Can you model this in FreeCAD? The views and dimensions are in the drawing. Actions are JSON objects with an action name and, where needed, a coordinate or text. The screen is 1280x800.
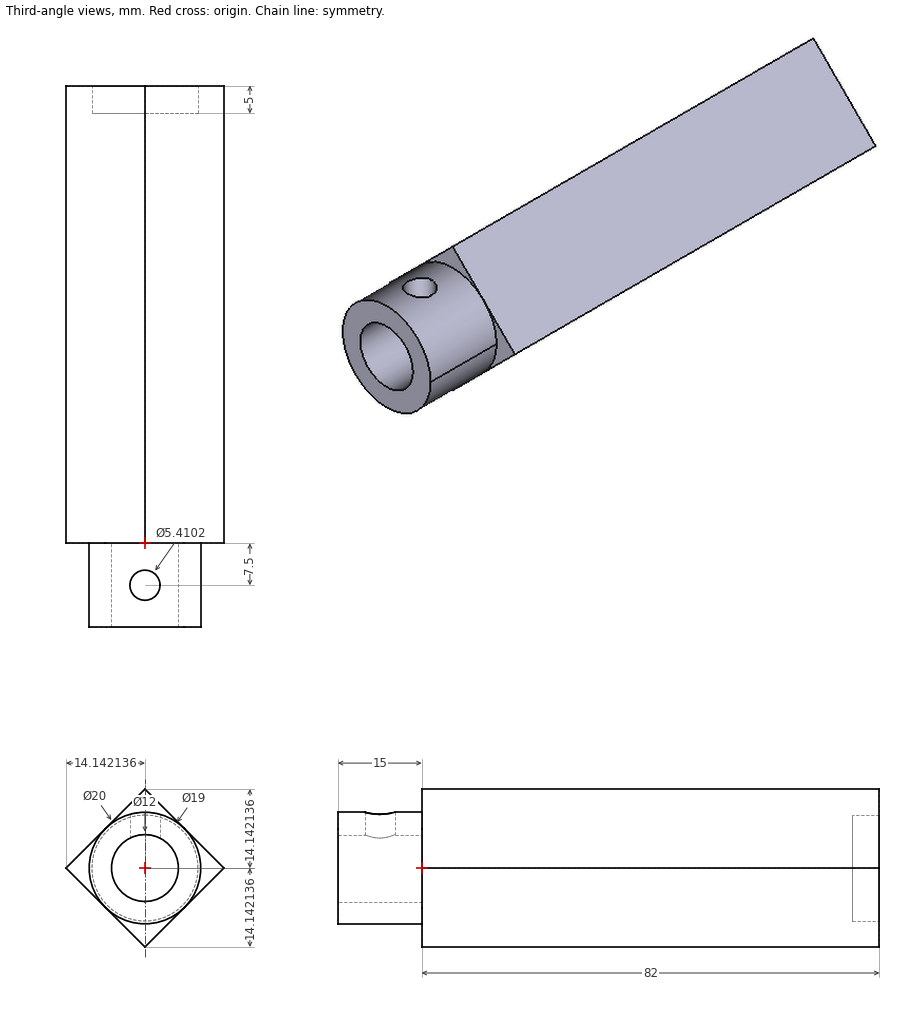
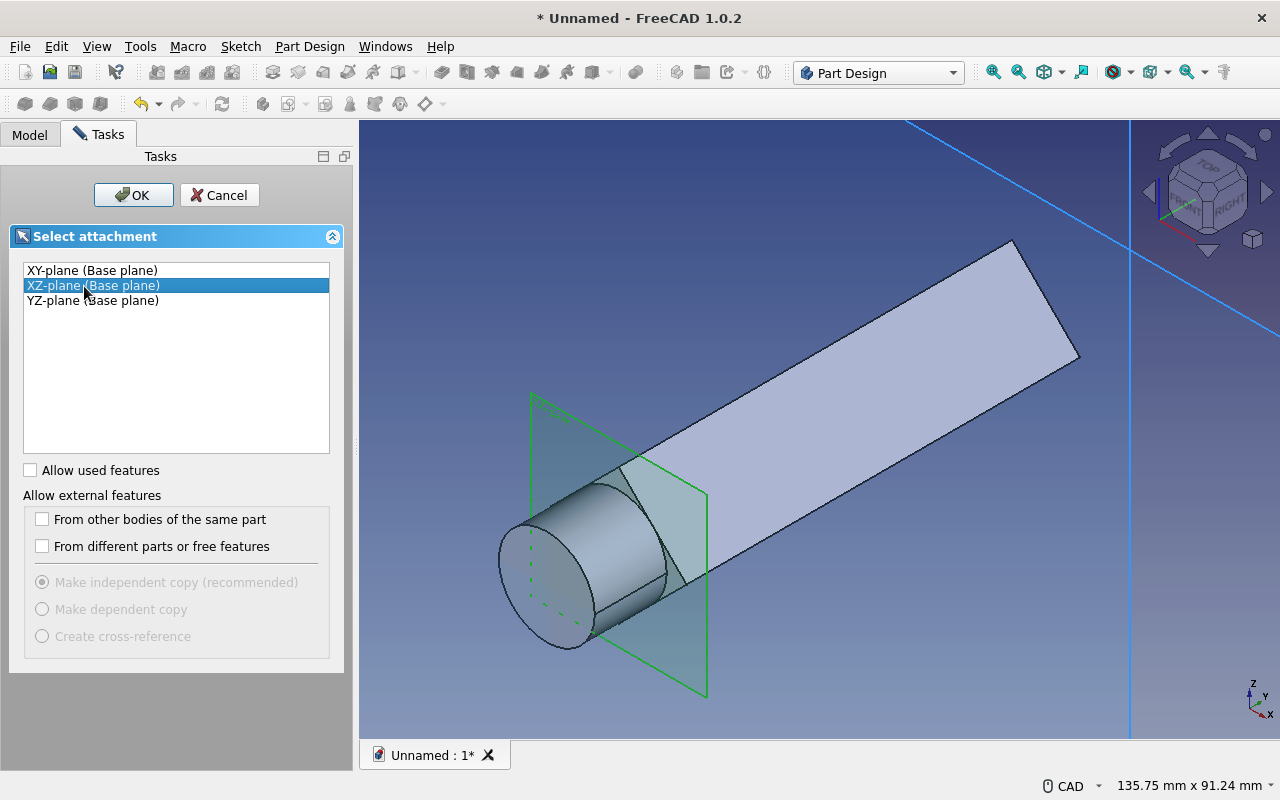
{"action": "left_click", "coordinate": [134, 195]}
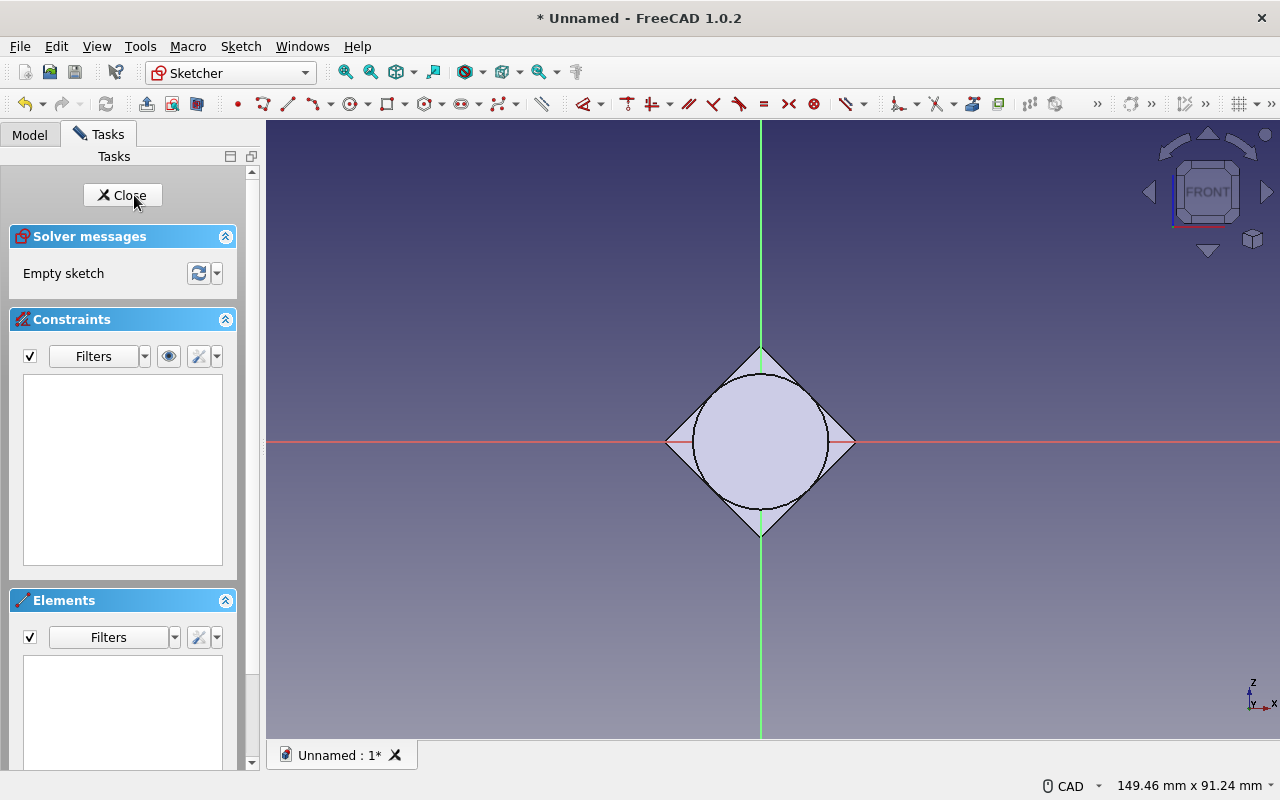
{"action": "key", "text": "q s"}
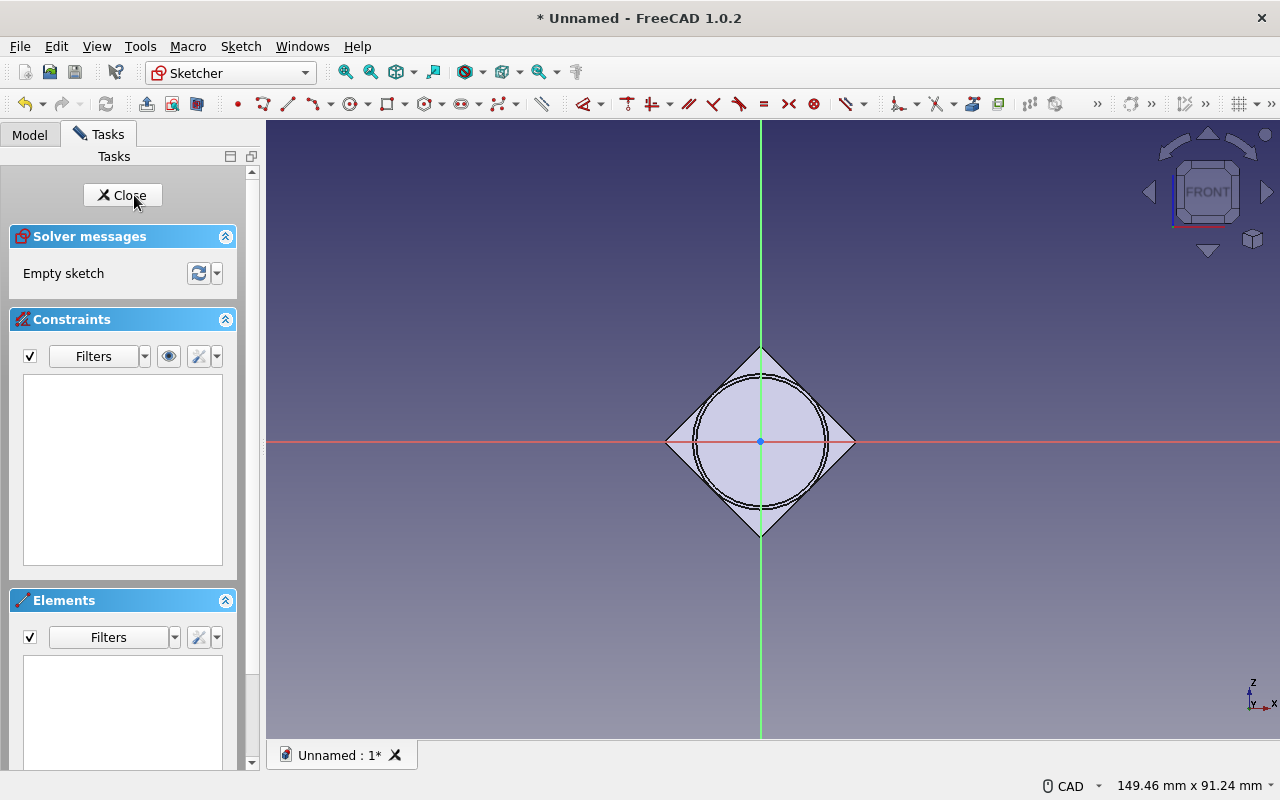
{"action": "scroll", "coordinate": [775, 445], "scroll_direction": "up", "scroll_amount": 8}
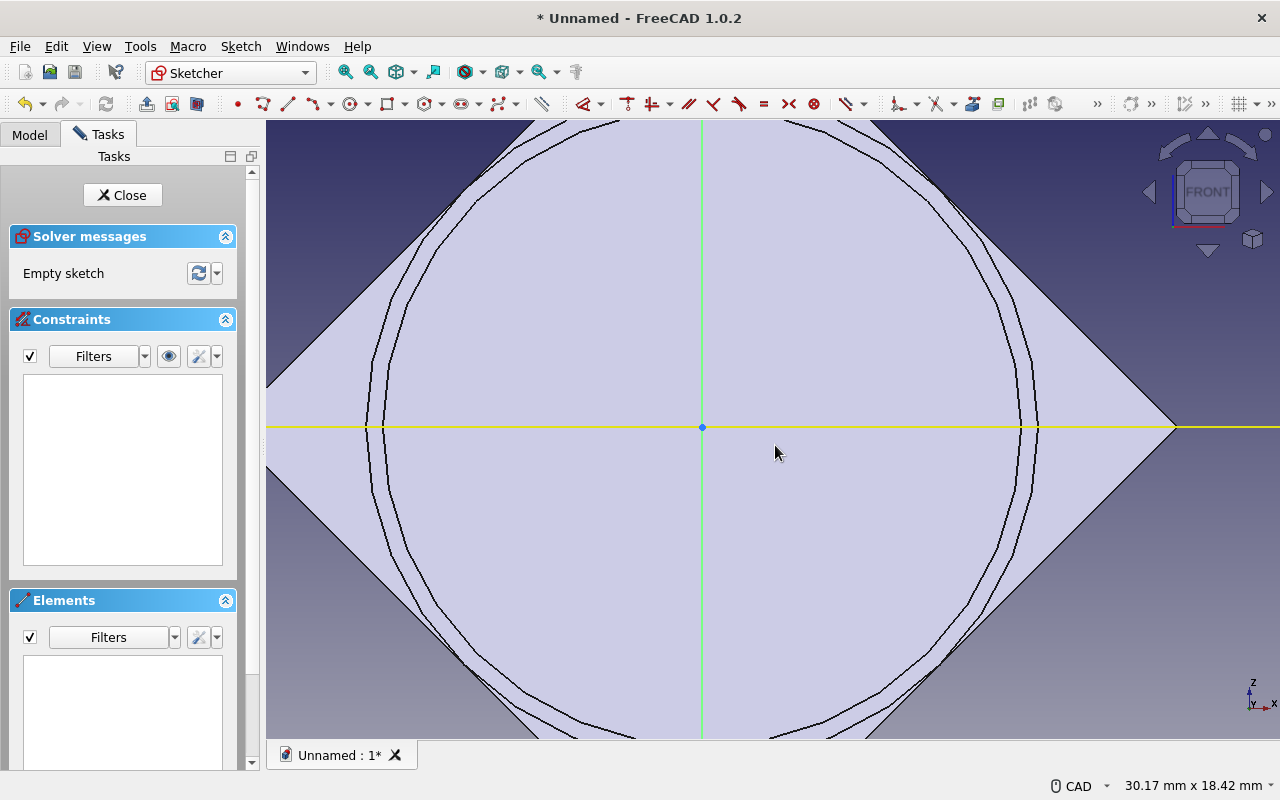
{"action": "key", "text": "g c"}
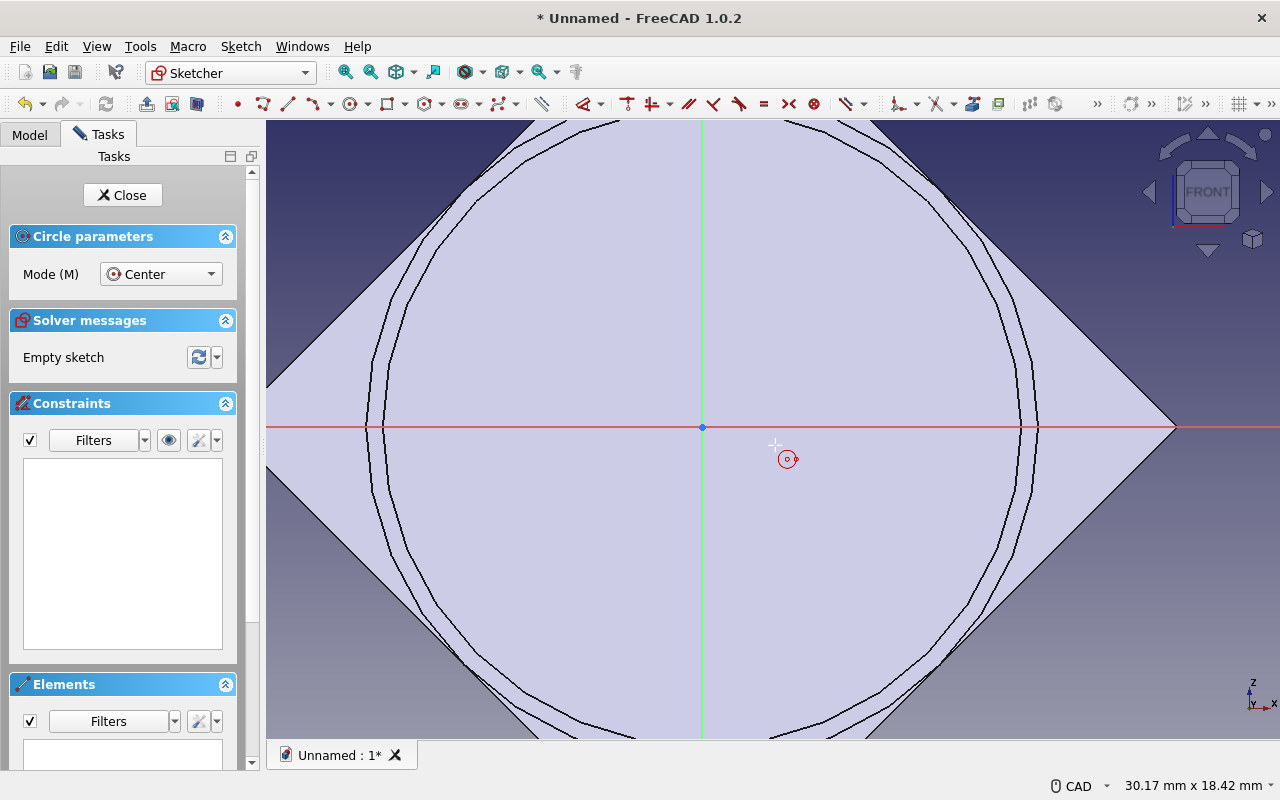
{"action": "left_click", "coordinate": [702, 427]}
{"action": "mouse_move", "coordinate": [845, 285]}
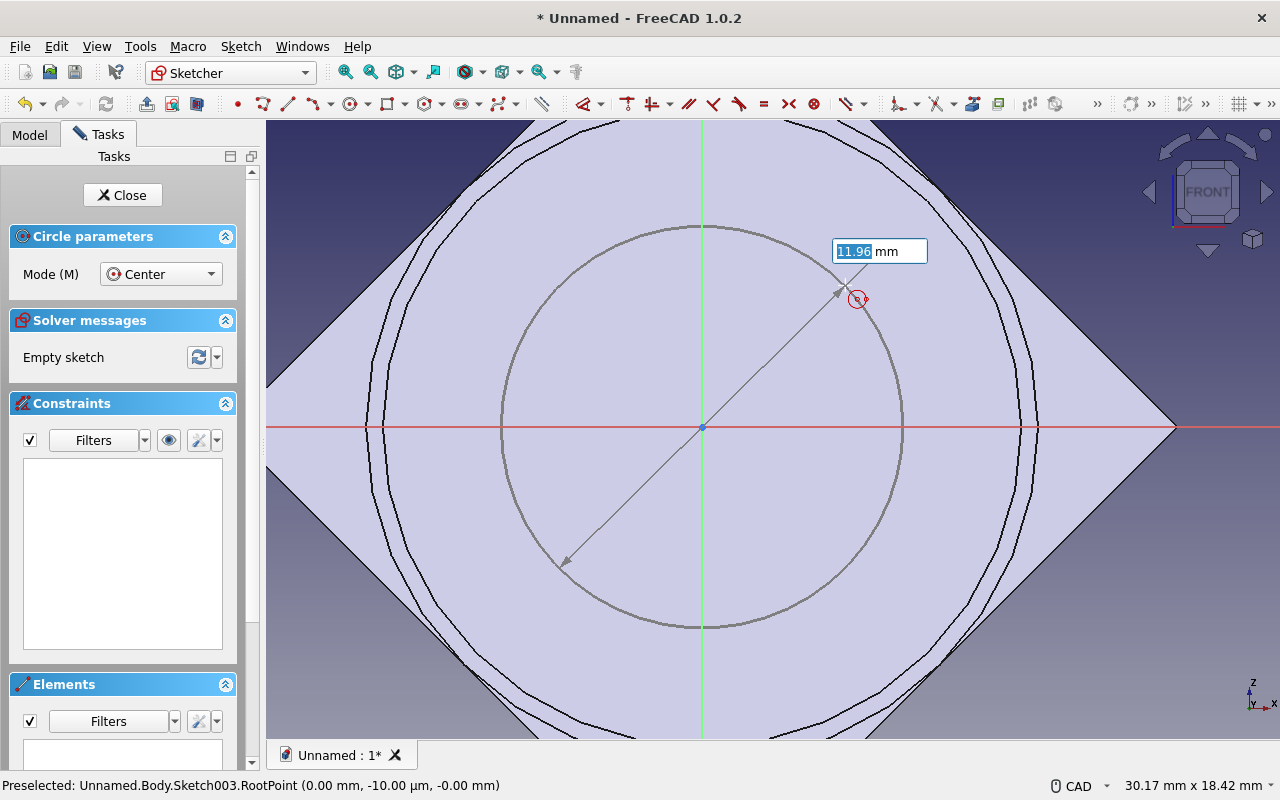
{"action": "type", "text": "12"}
{"action": "key", "text": "Return"}
{"action": "key", "text": "Escape"}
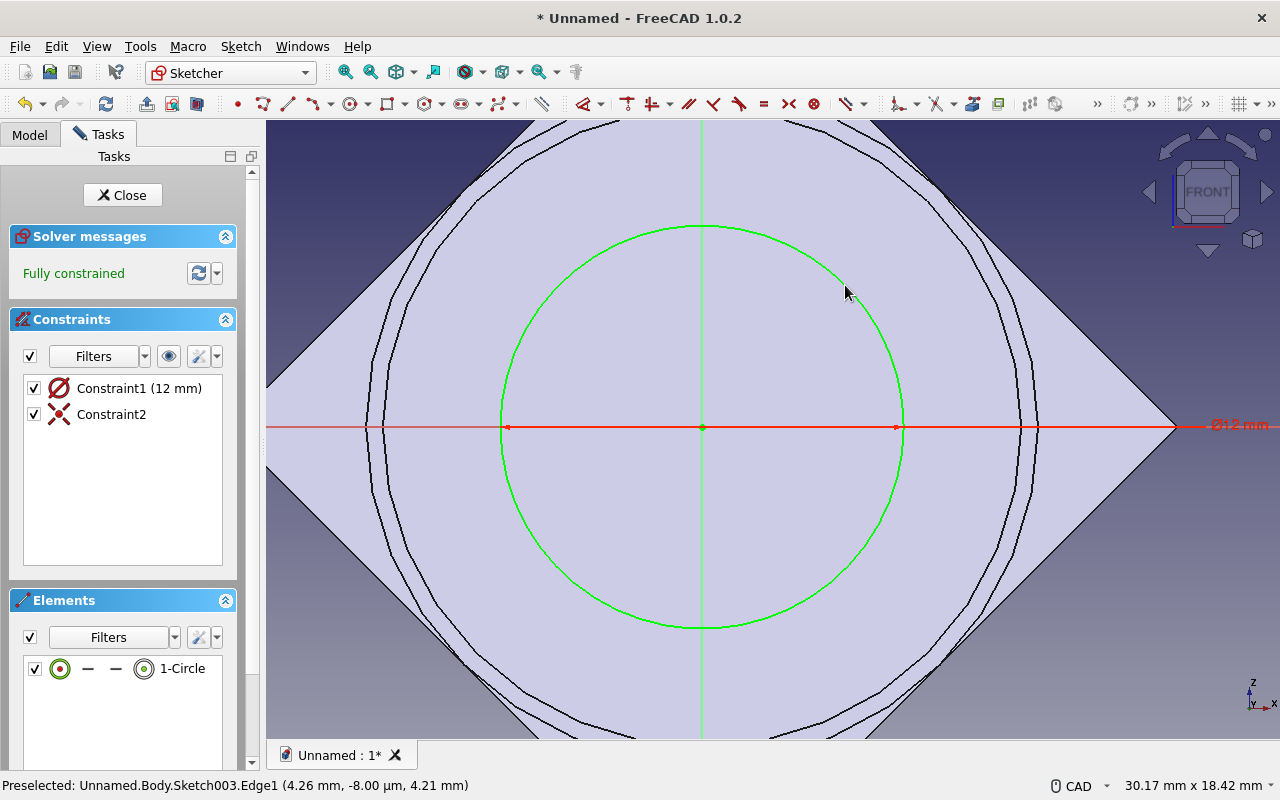
{"action": "left_click", "coordinate": [123, 195]}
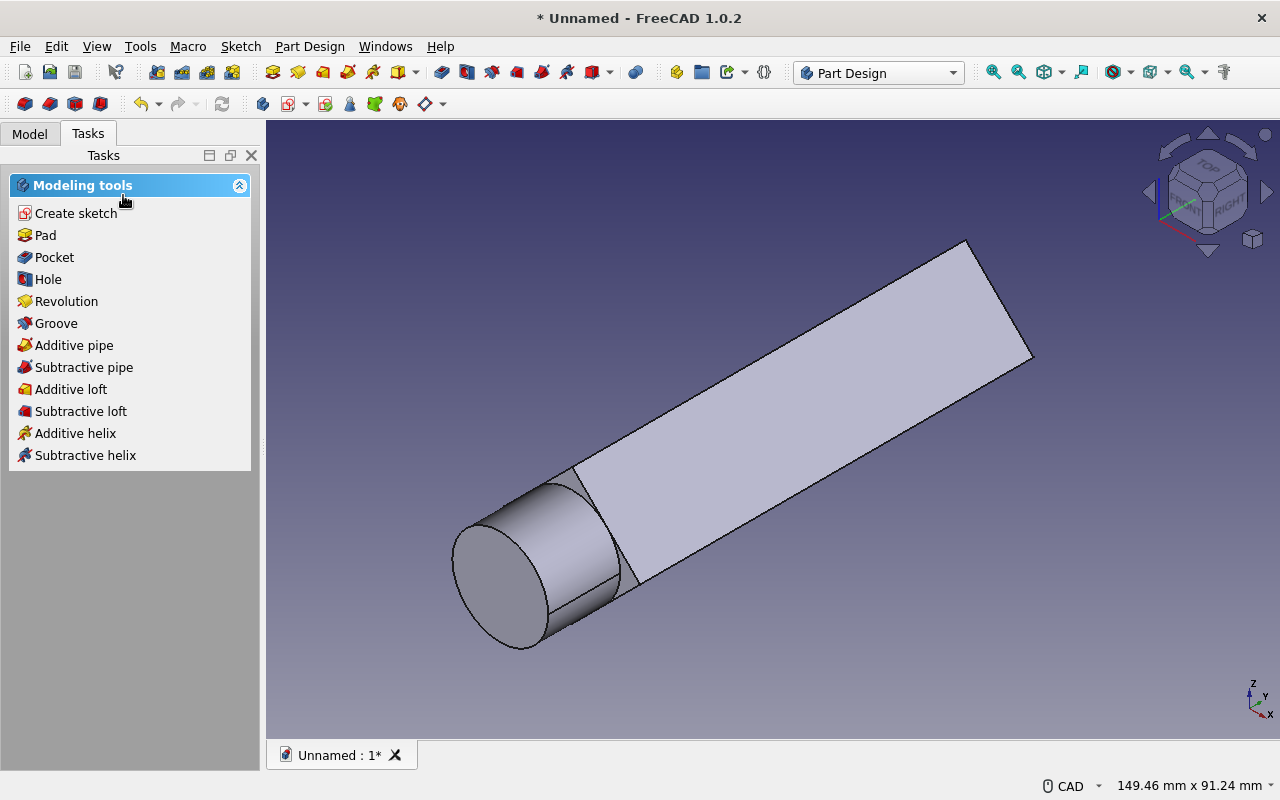
{"action": "left_click", "coordinate": [442, 72]}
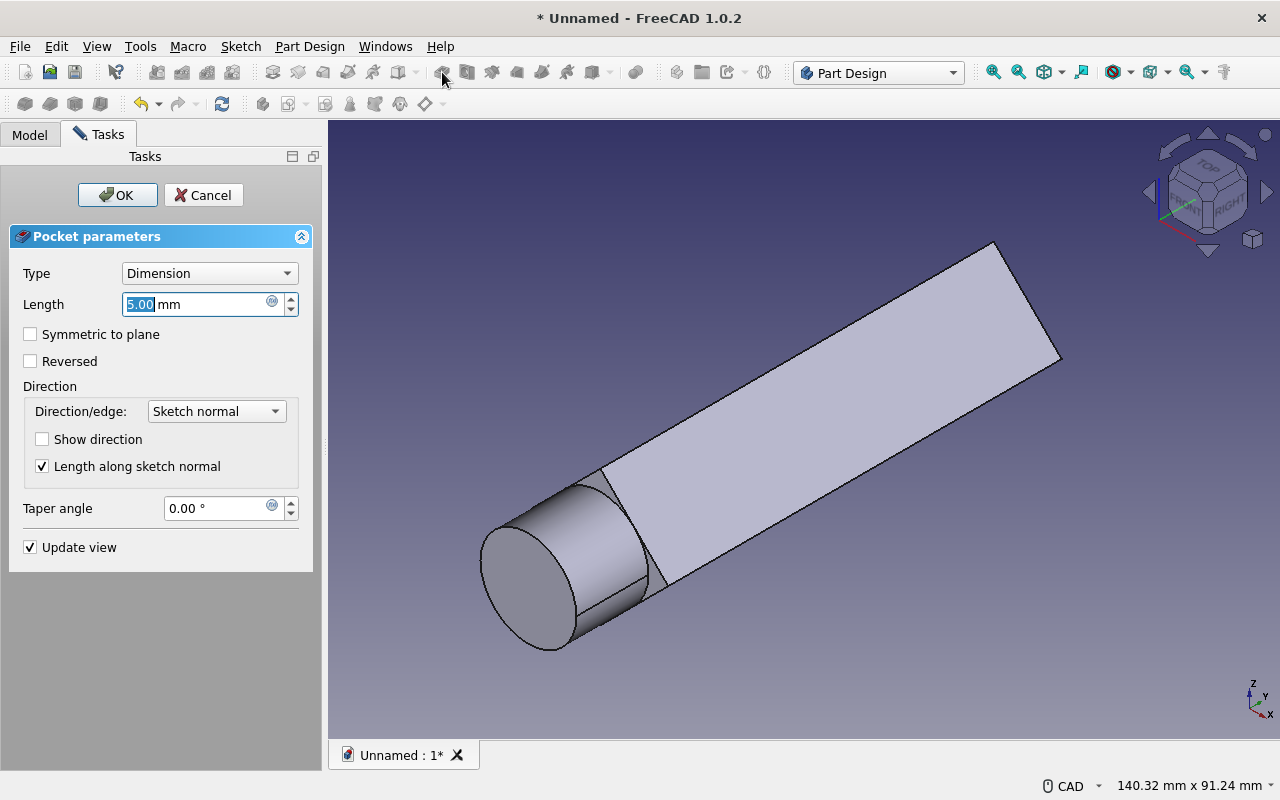
{"action": "left_click", "coordinate": [210, 274]}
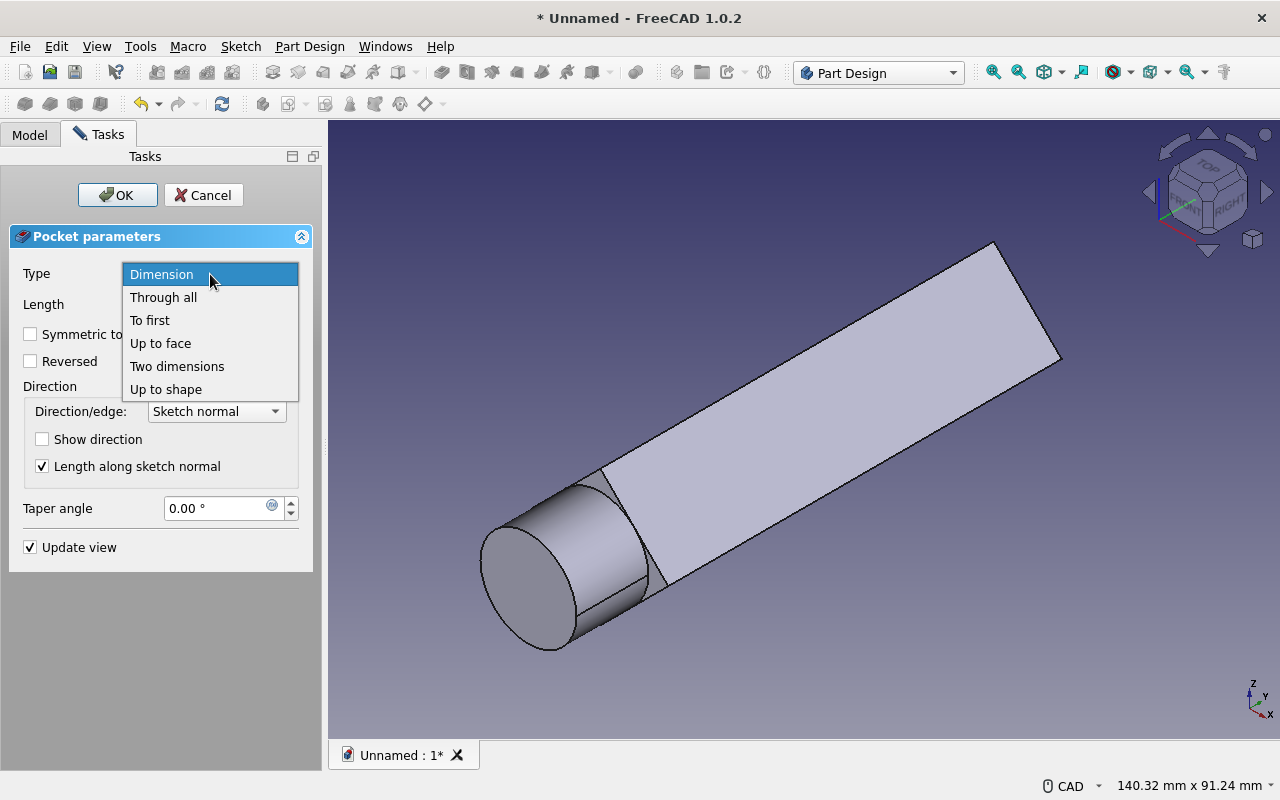
{"action": "left_click", "coordinate": [208, 298]}